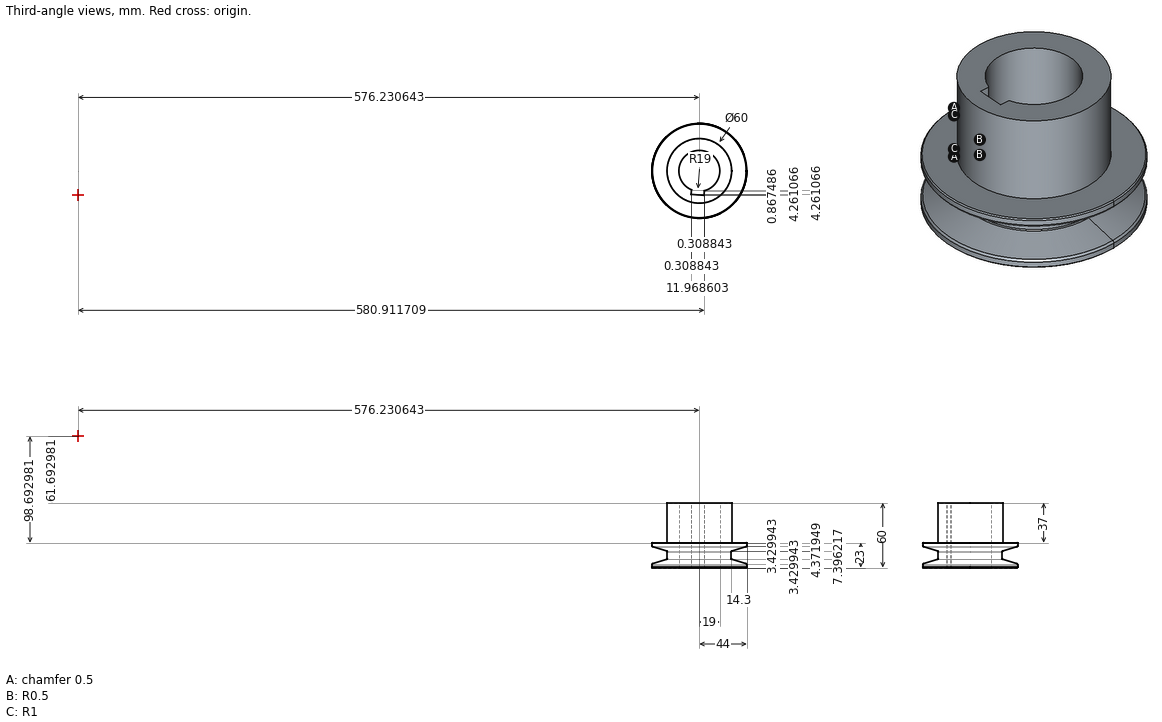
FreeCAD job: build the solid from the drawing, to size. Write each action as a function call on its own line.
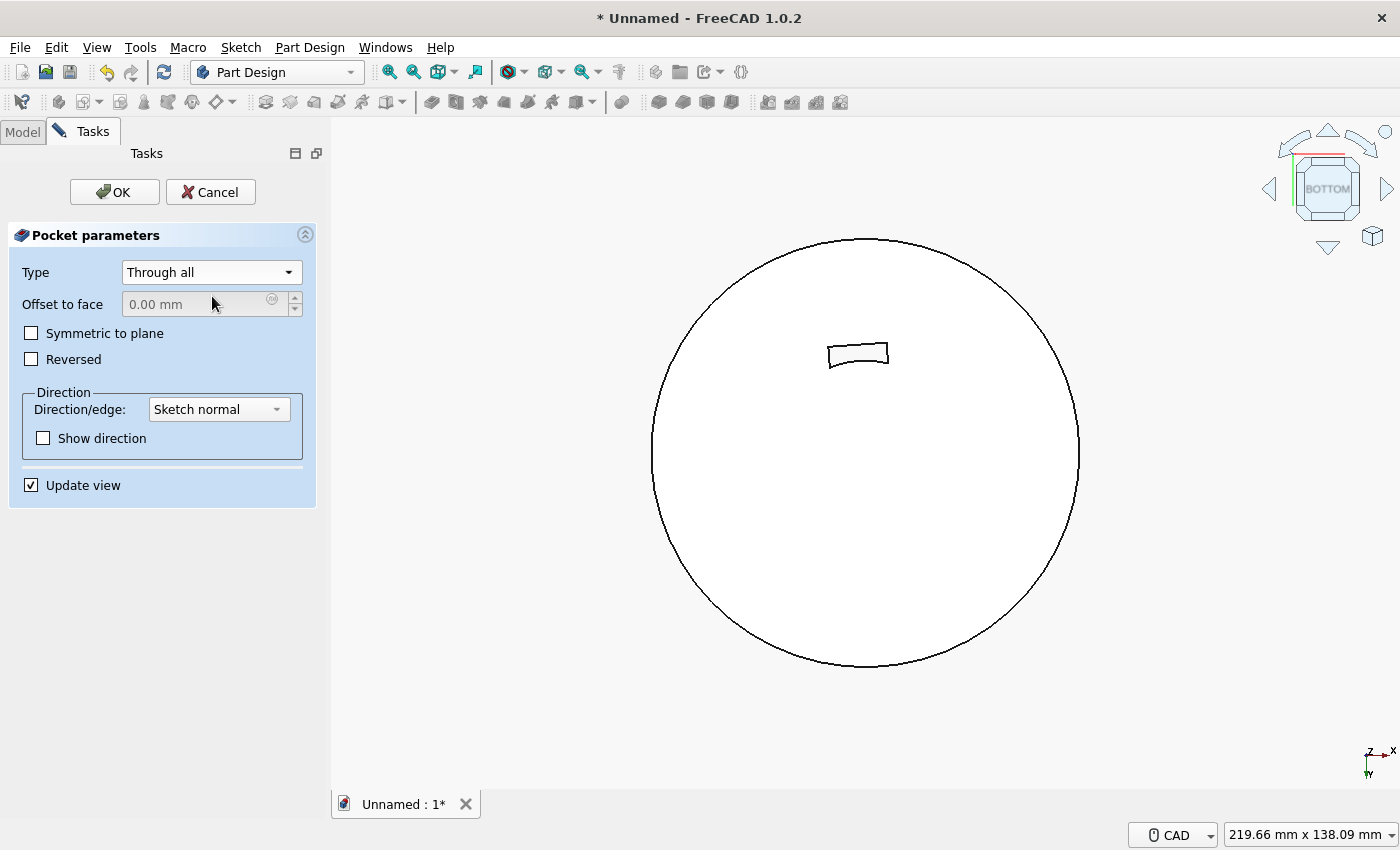
click(115, 192)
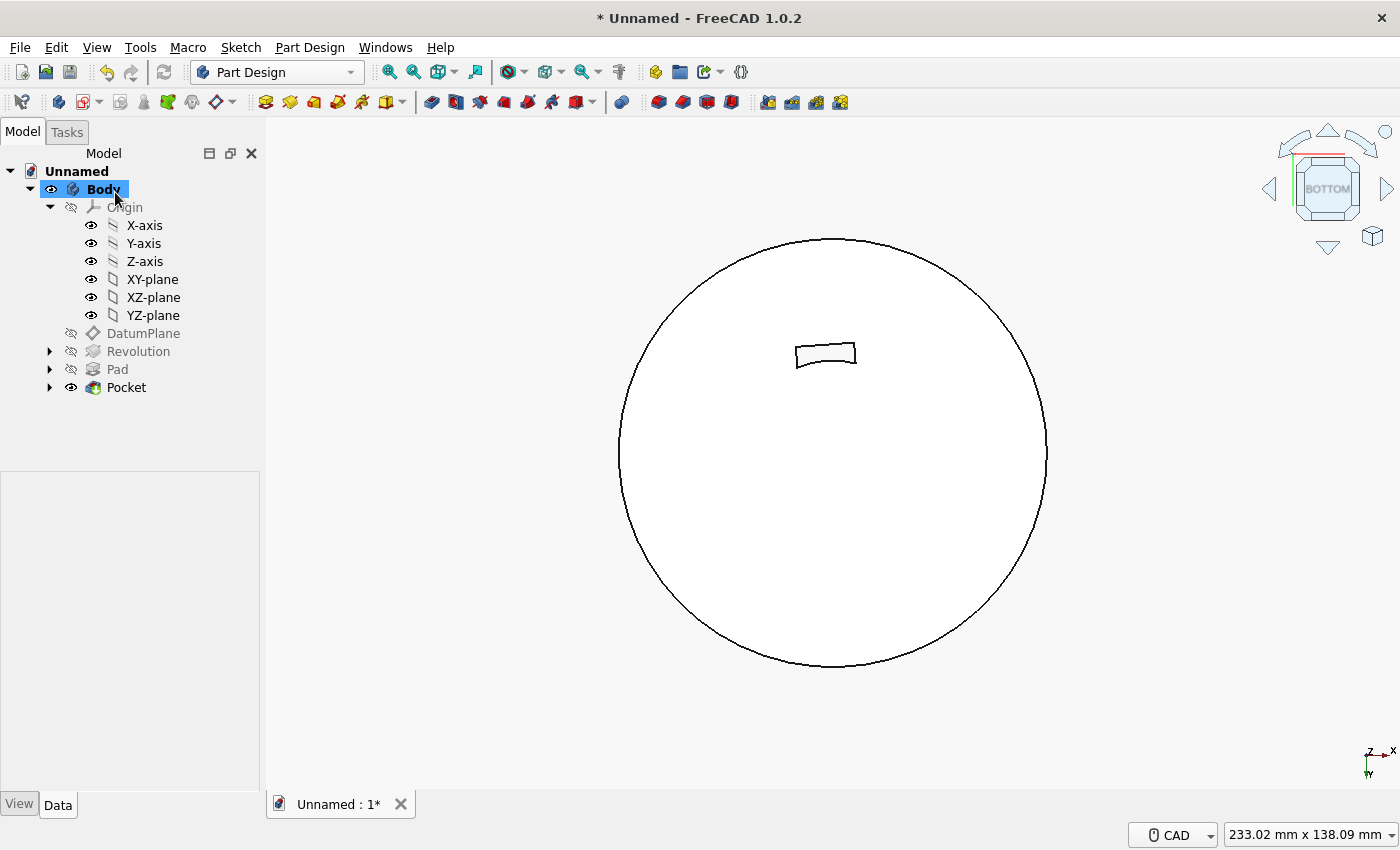
click(136, 297)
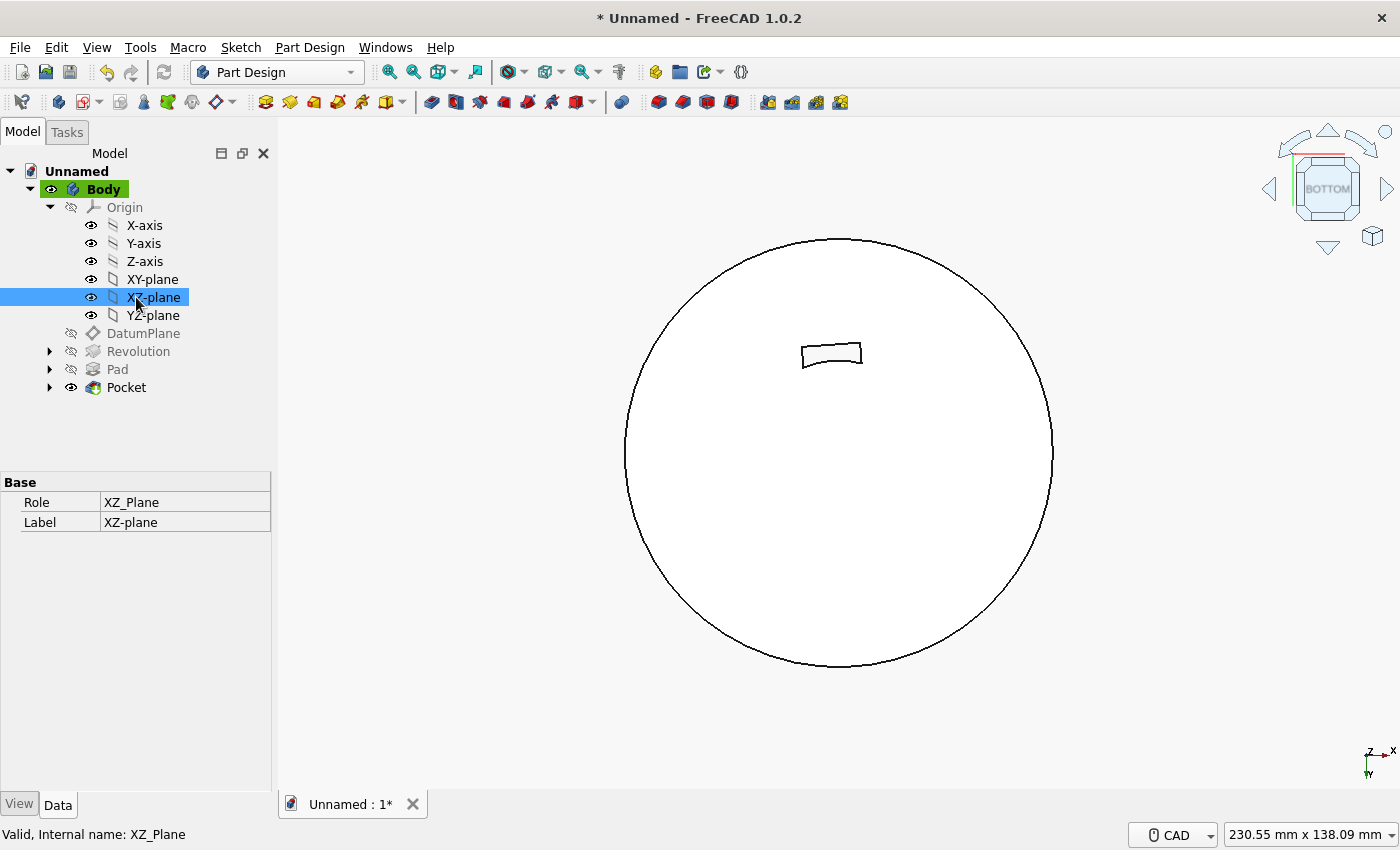
click(216, 102)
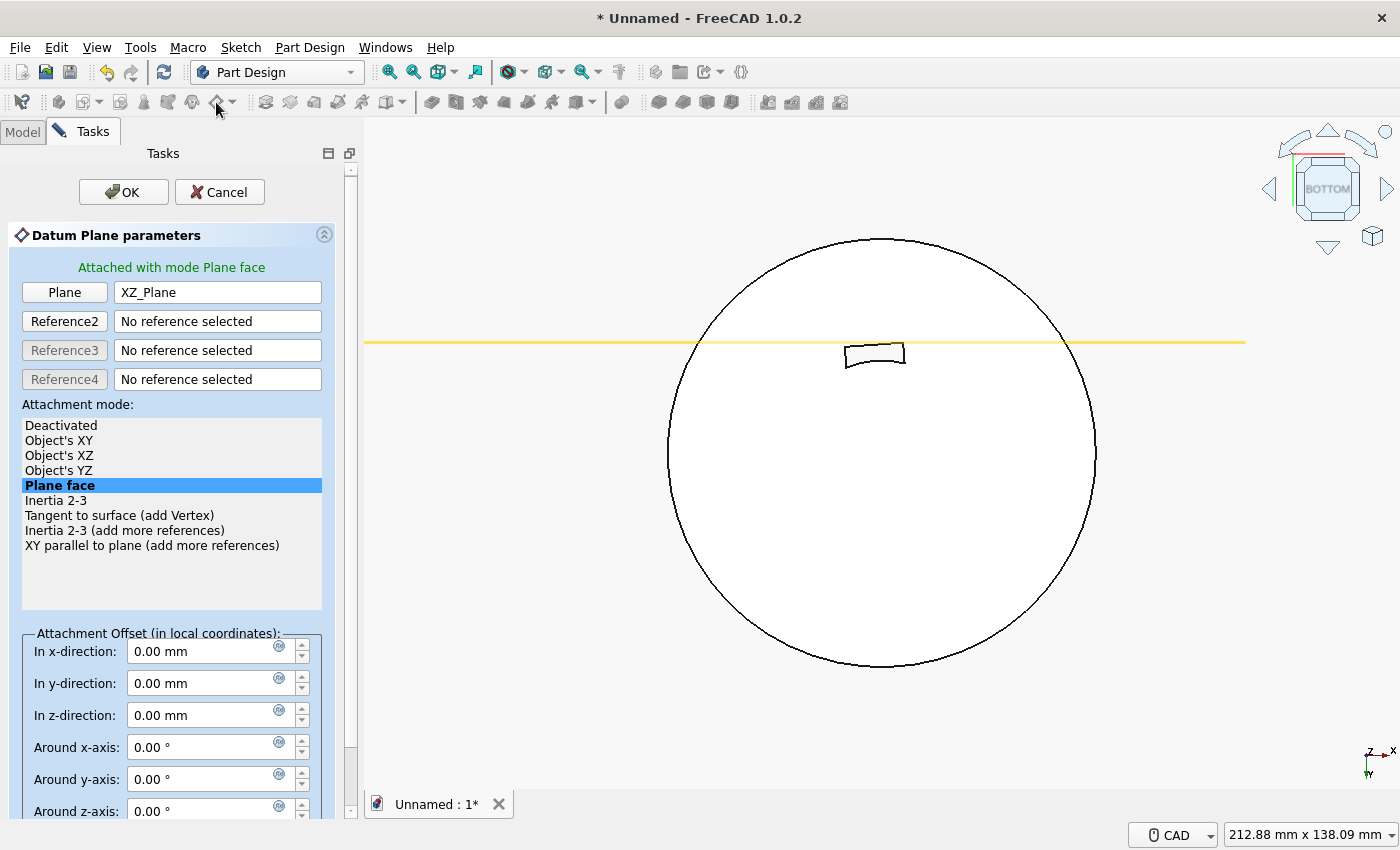
triple_click(210, 715)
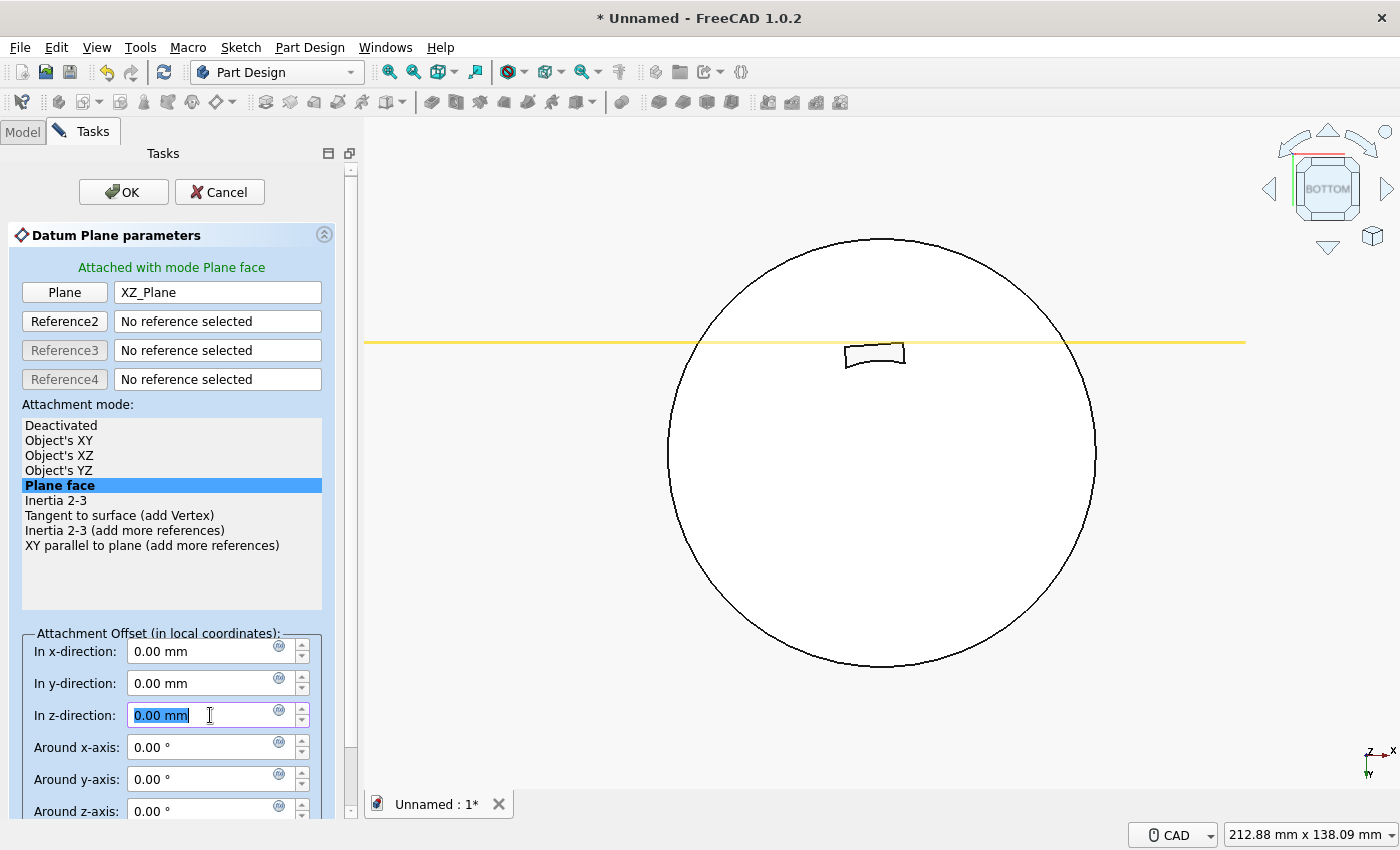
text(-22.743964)
key(Tab)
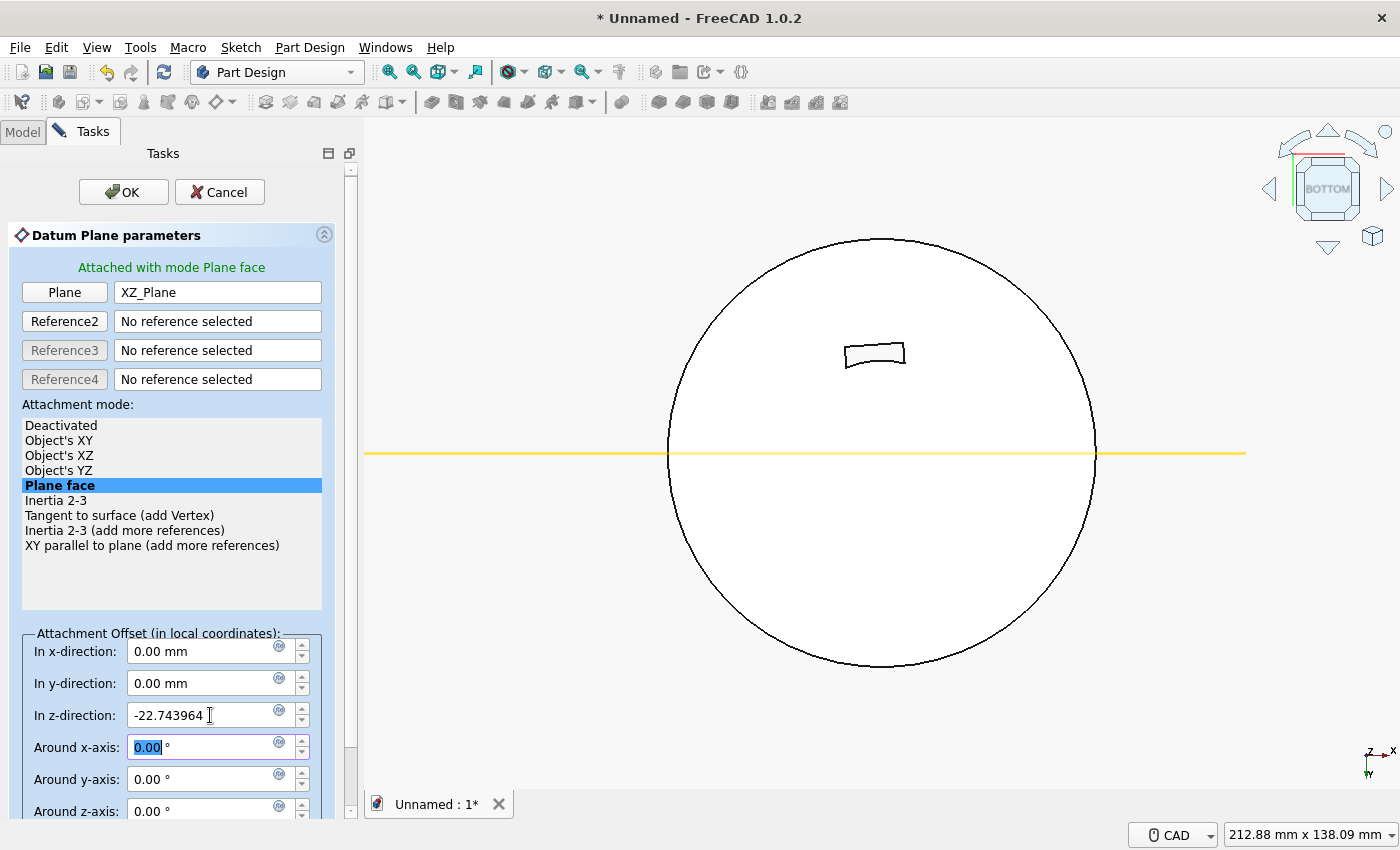
click(124, 192)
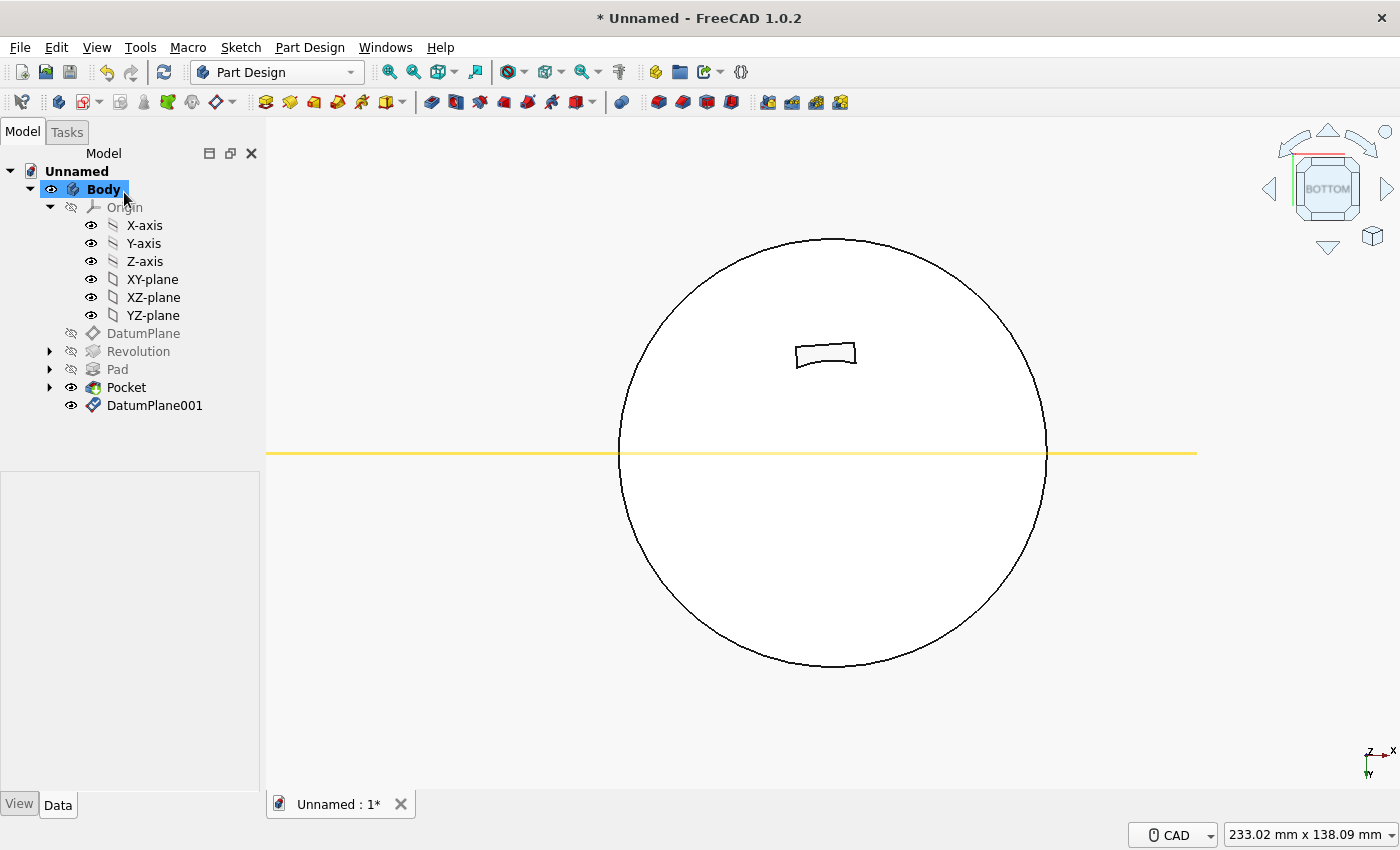
click(116, 405)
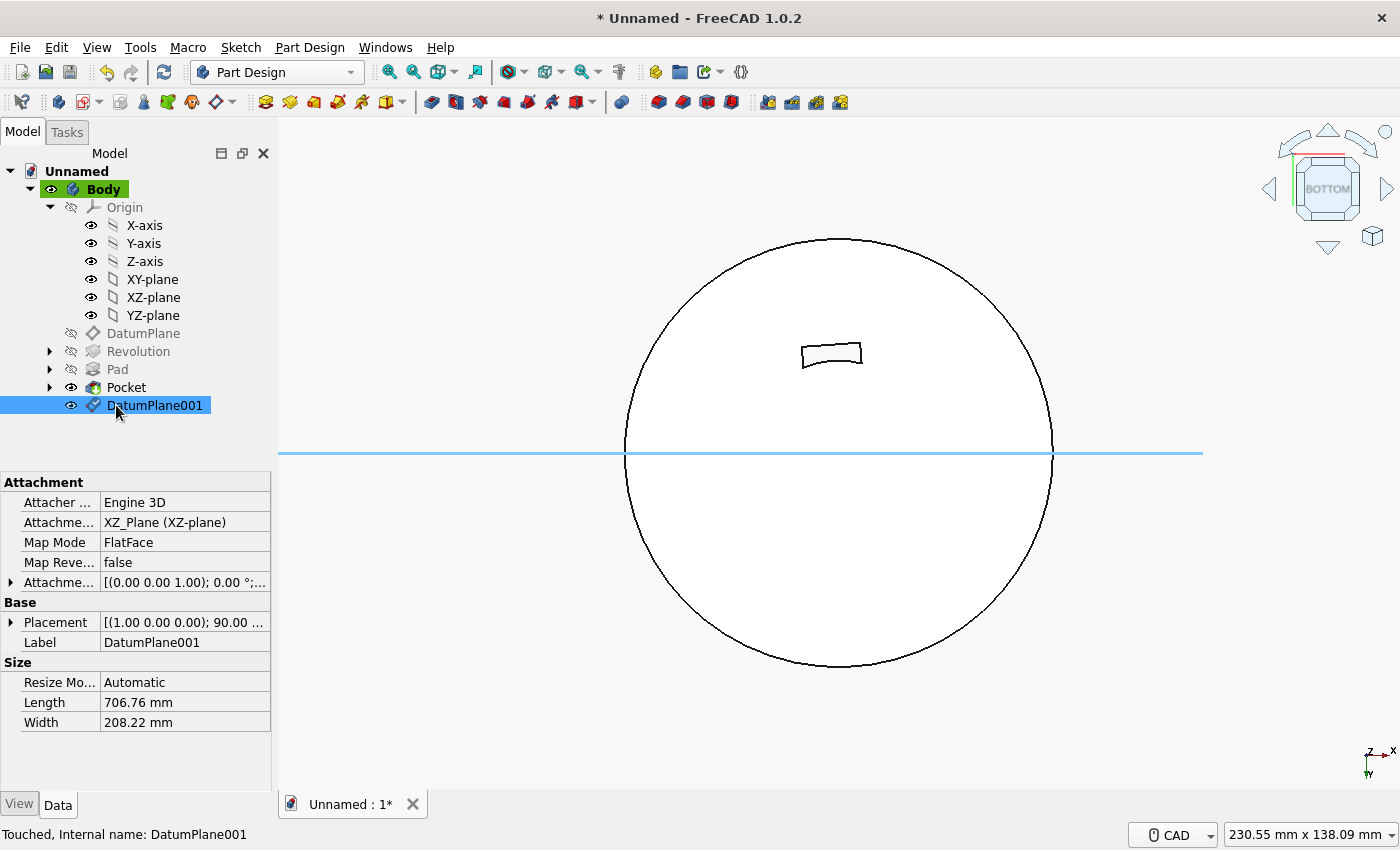
click(84, 102)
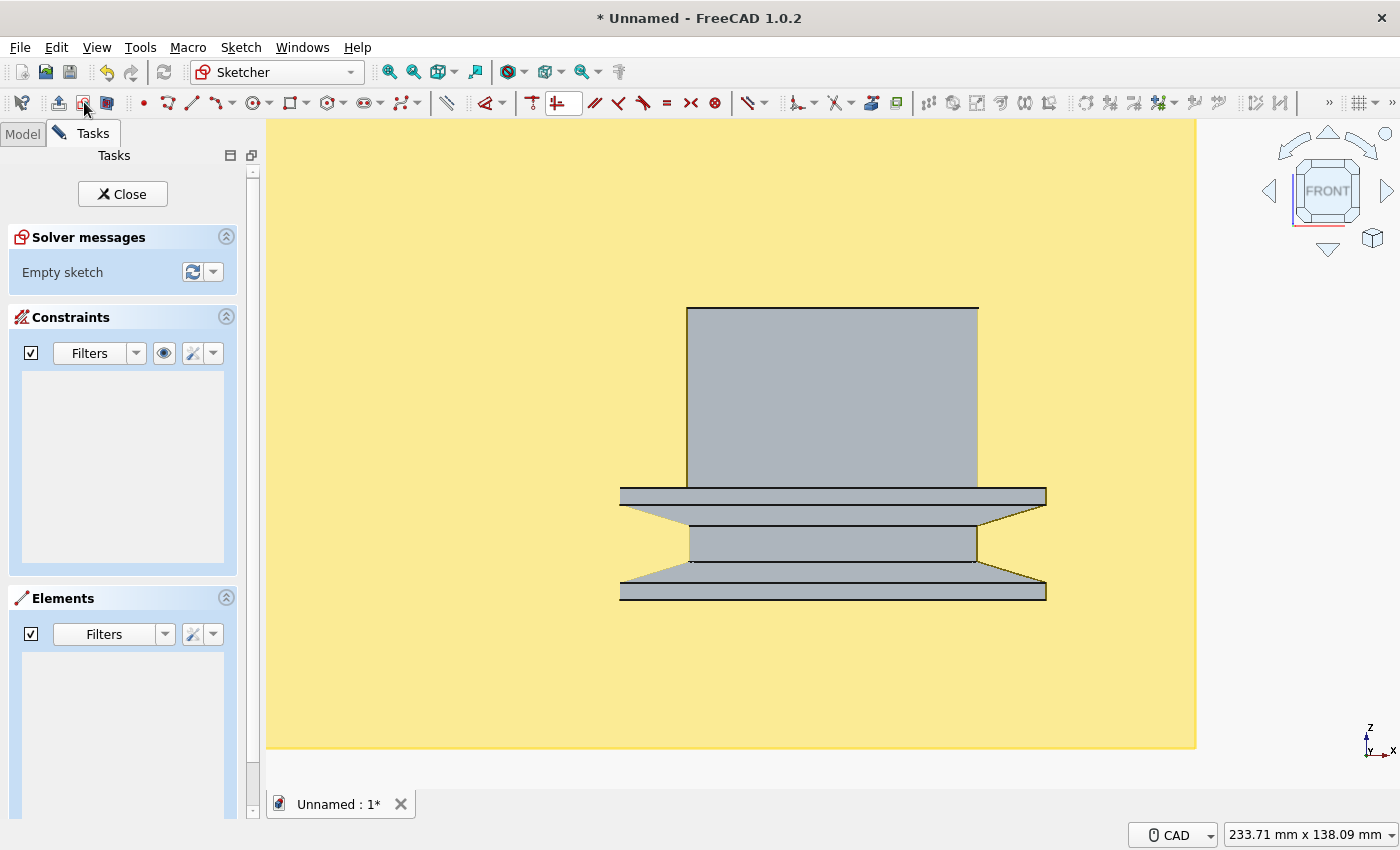
key(q)
key(s)